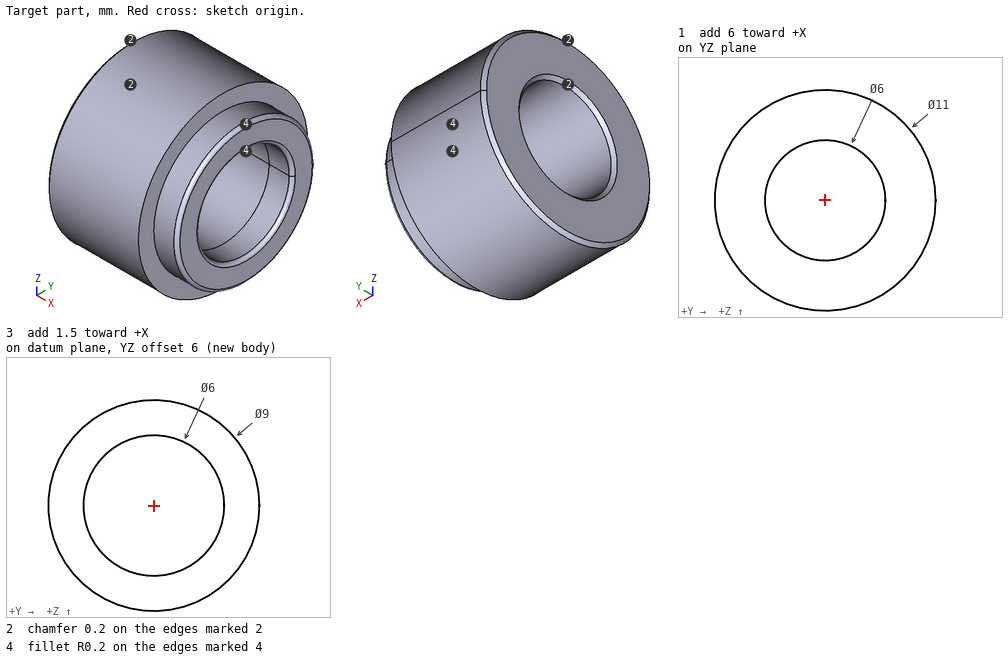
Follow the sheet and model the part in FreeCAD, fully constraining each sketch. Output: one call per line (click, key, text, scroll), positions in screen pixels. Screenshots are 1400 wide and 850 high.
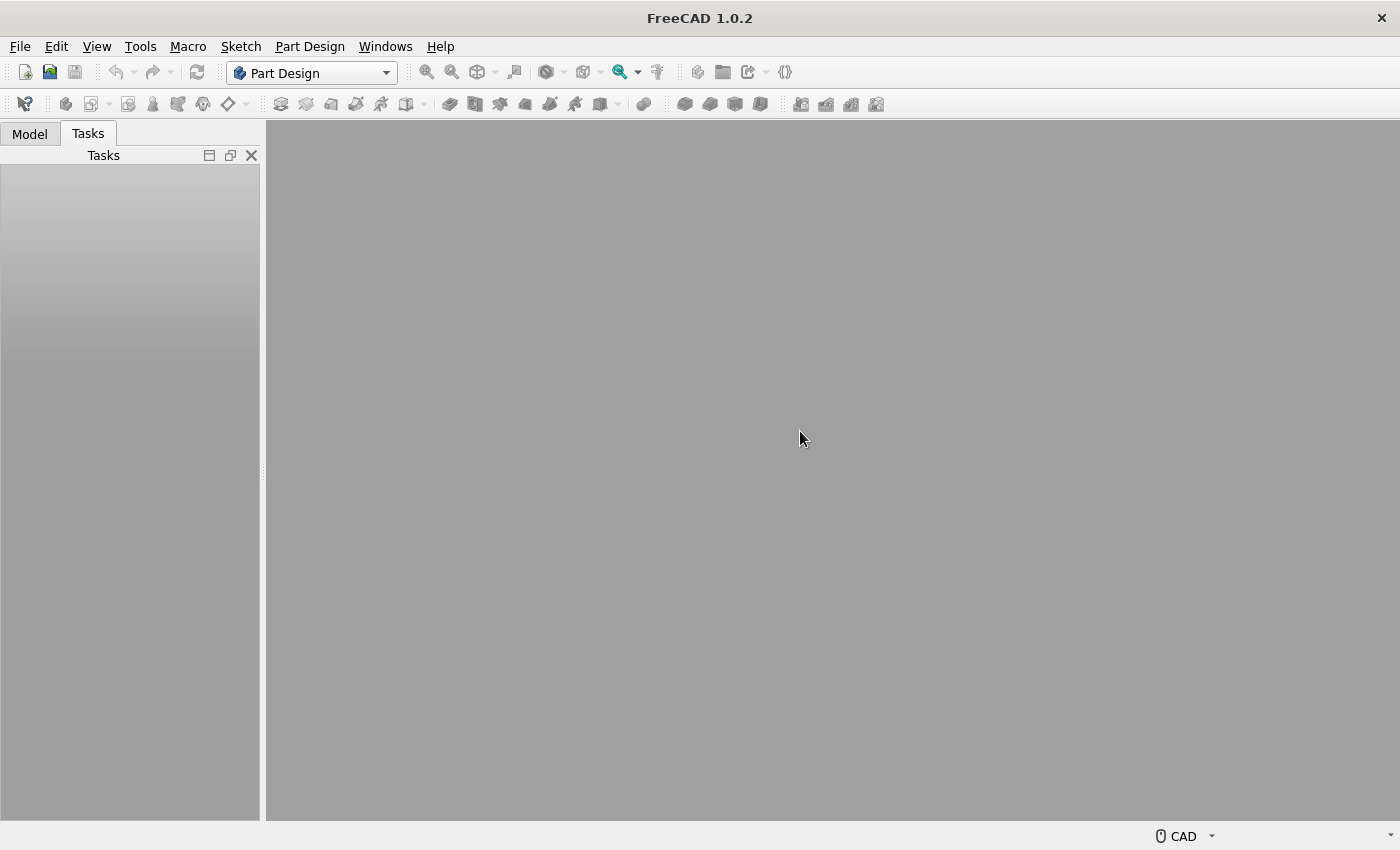
click(25, 72)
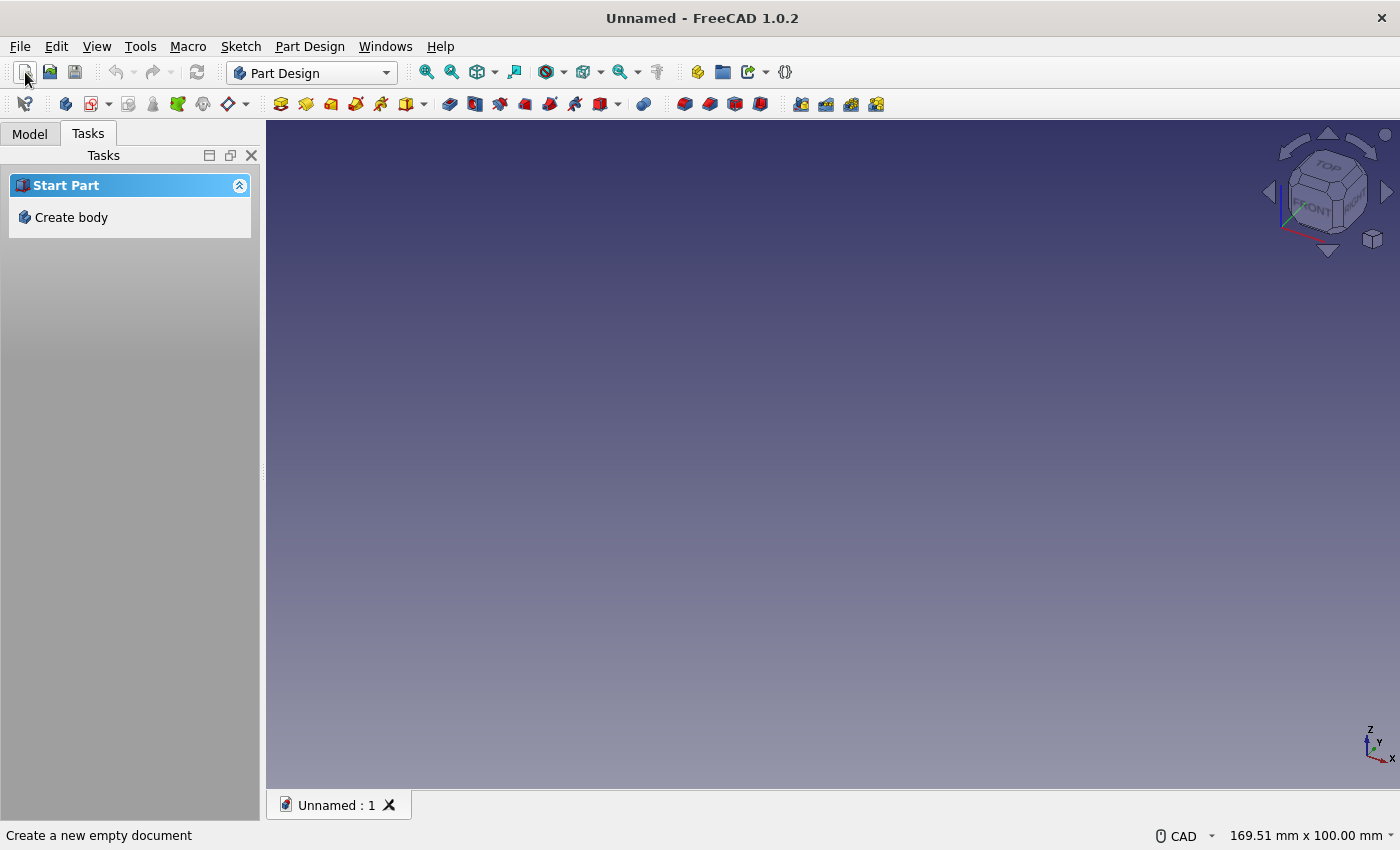
click(90, 104)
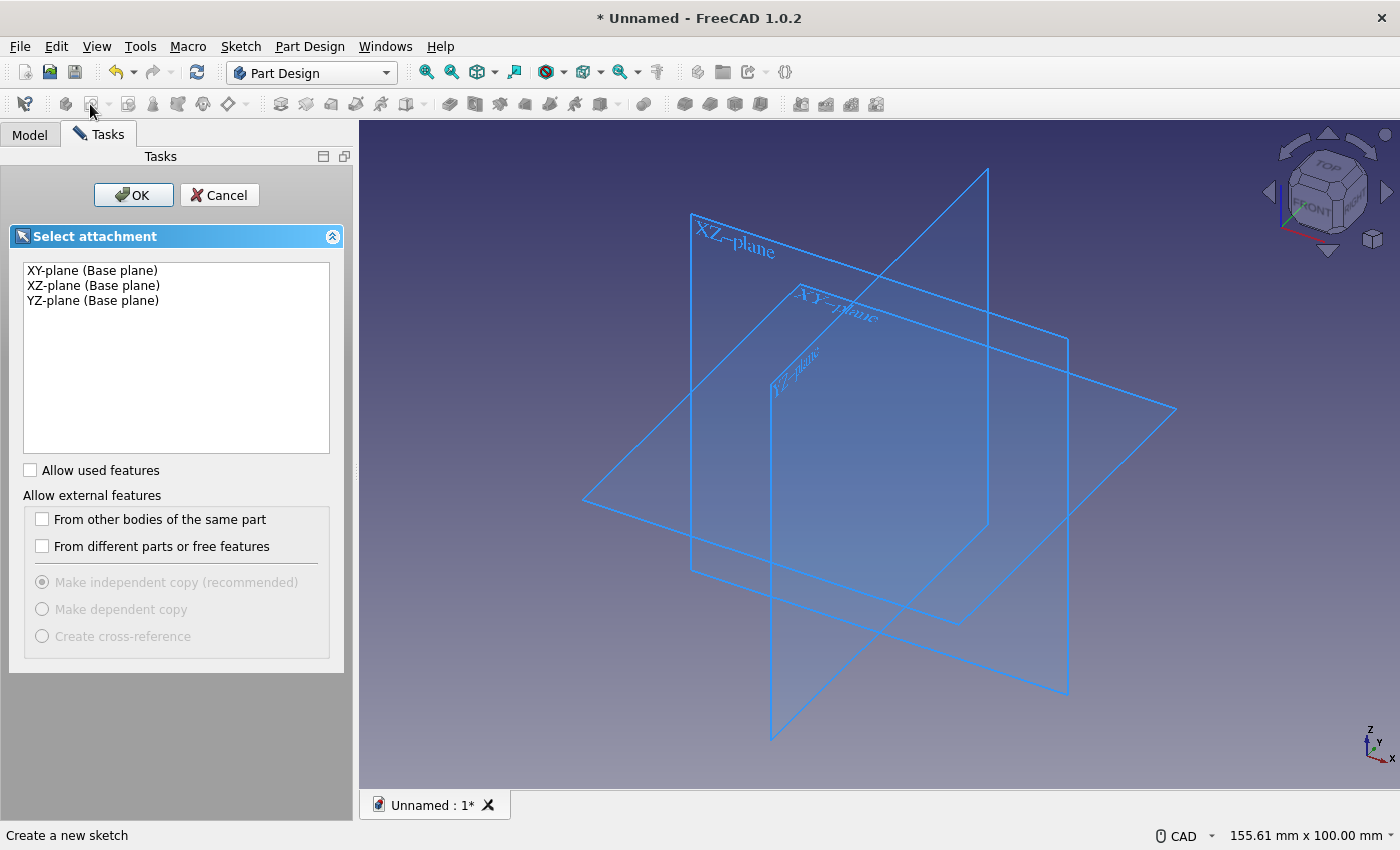
click(84, 300)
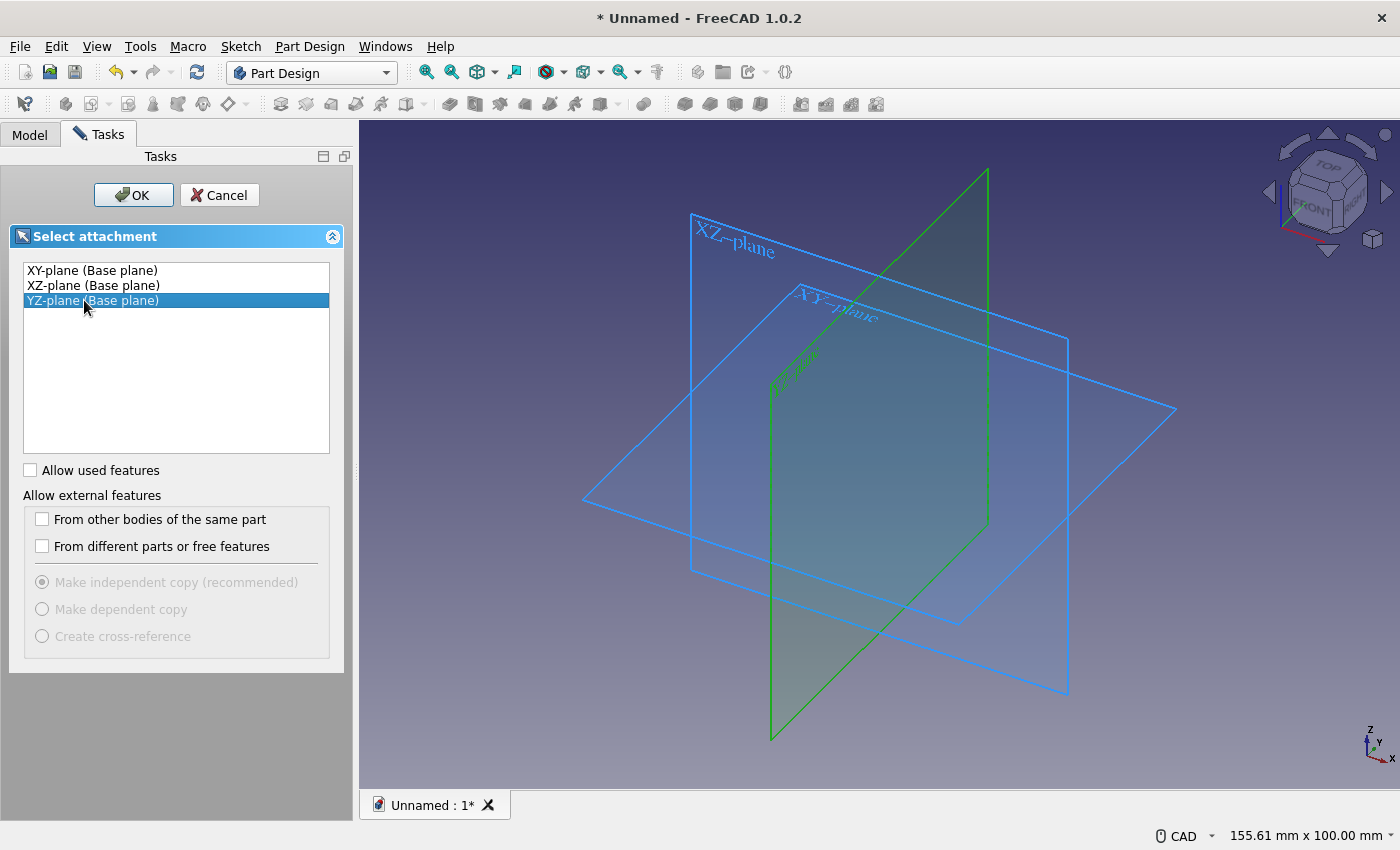
click(134, 195)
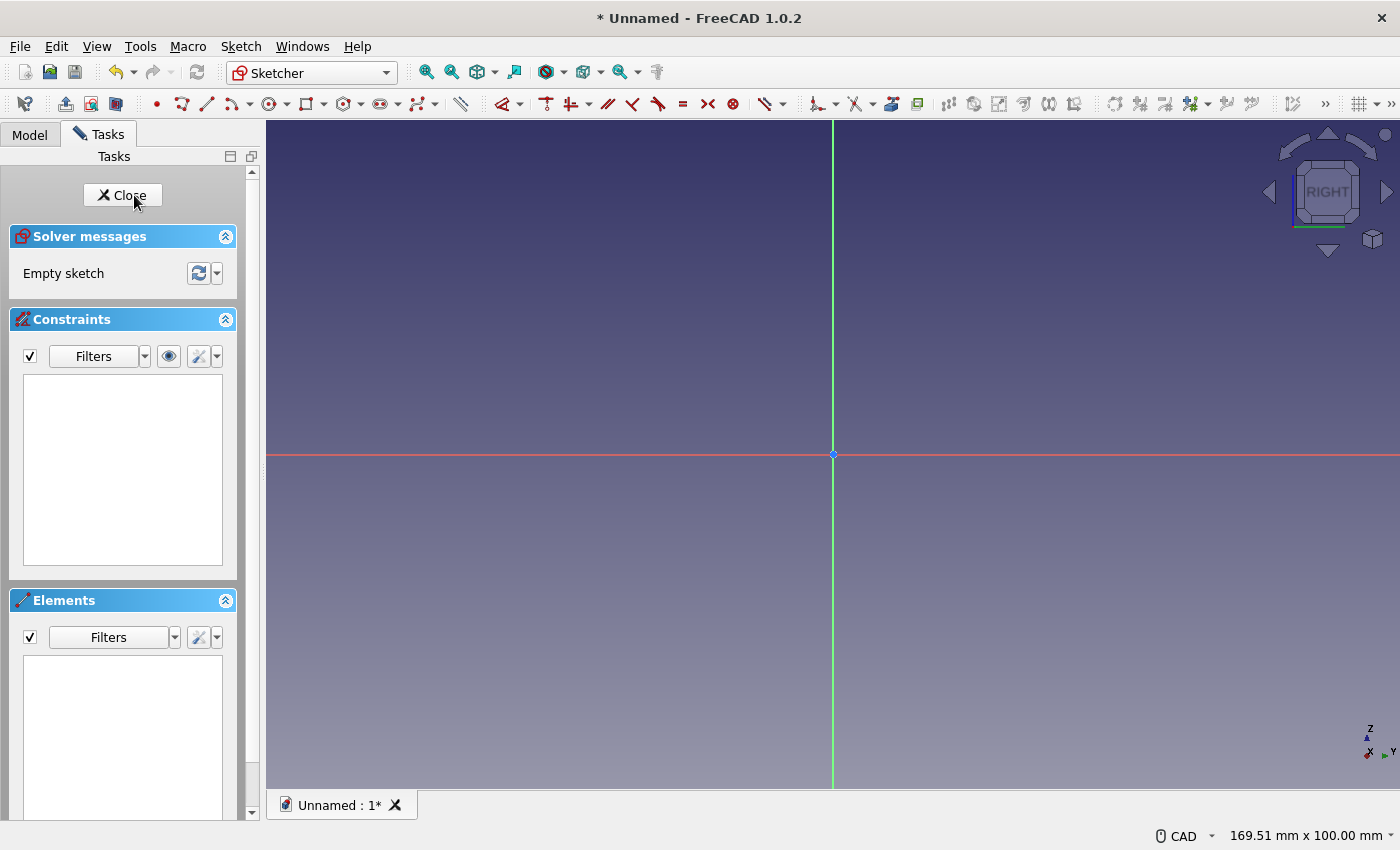
scroll(847, 455, up, 9)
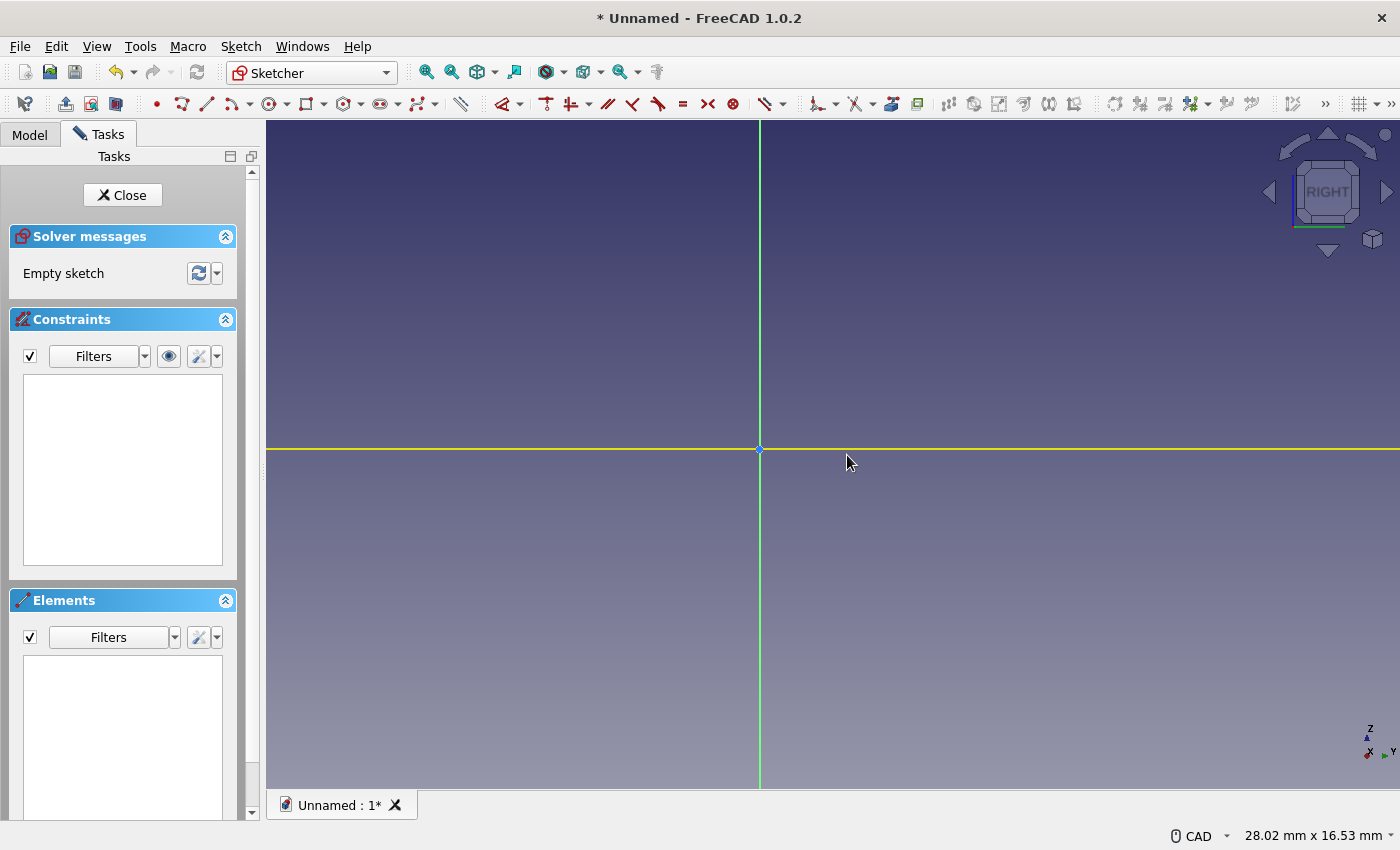
click(268, 104)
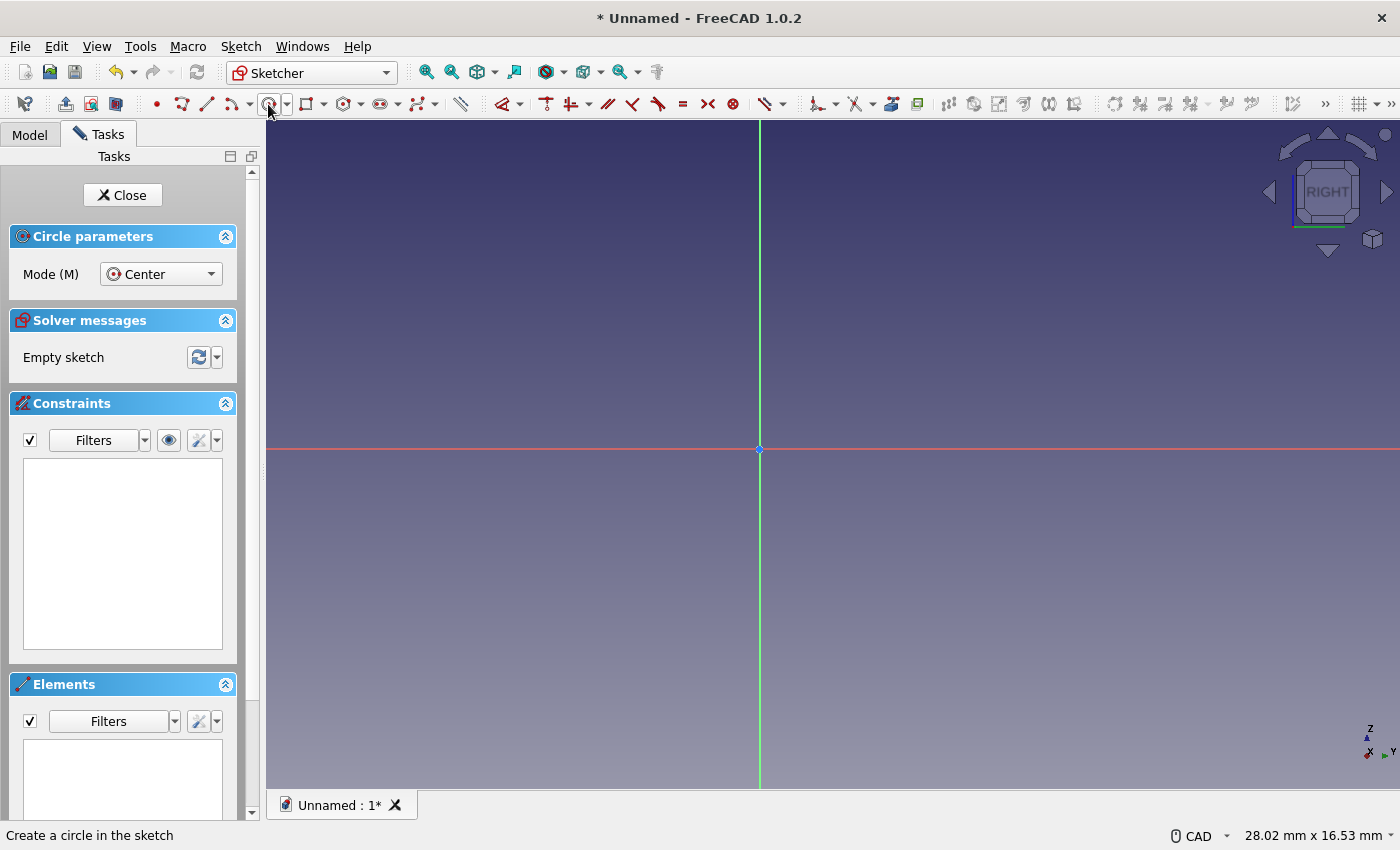
click(760, 449)
move(917, 292)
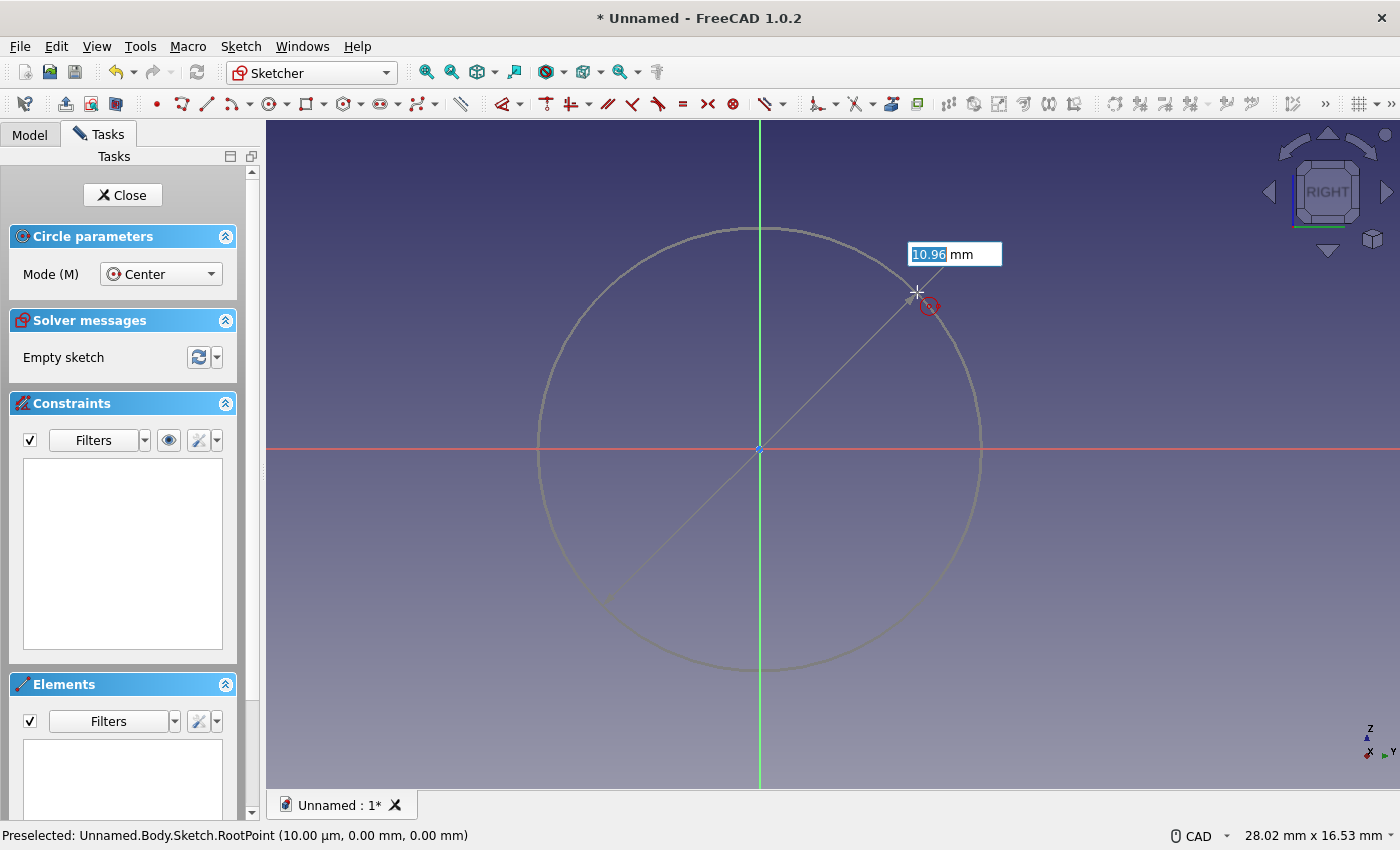
text(11)
key(Return)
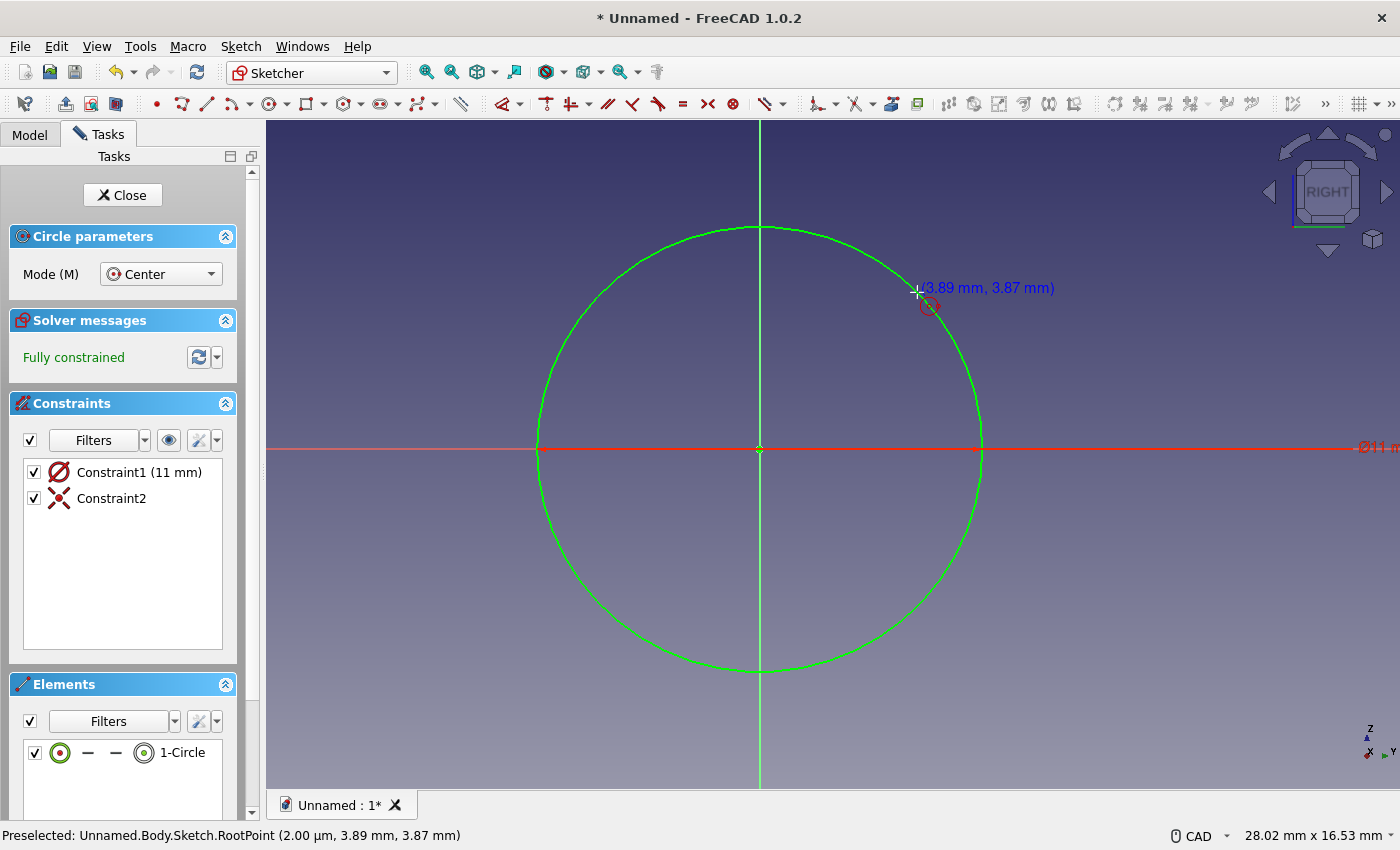
click(760, 449)
move(846, 364)